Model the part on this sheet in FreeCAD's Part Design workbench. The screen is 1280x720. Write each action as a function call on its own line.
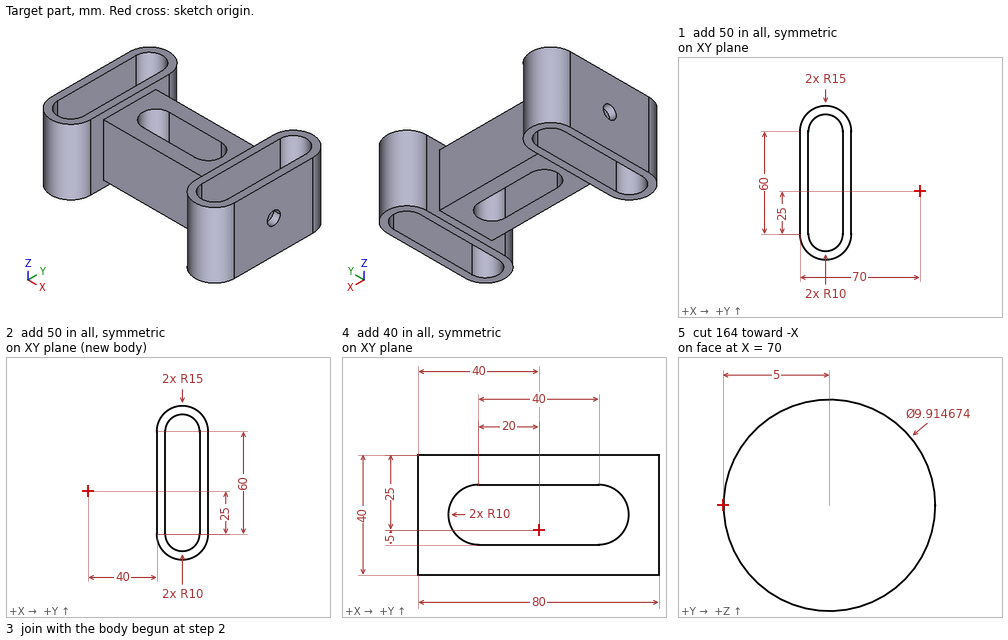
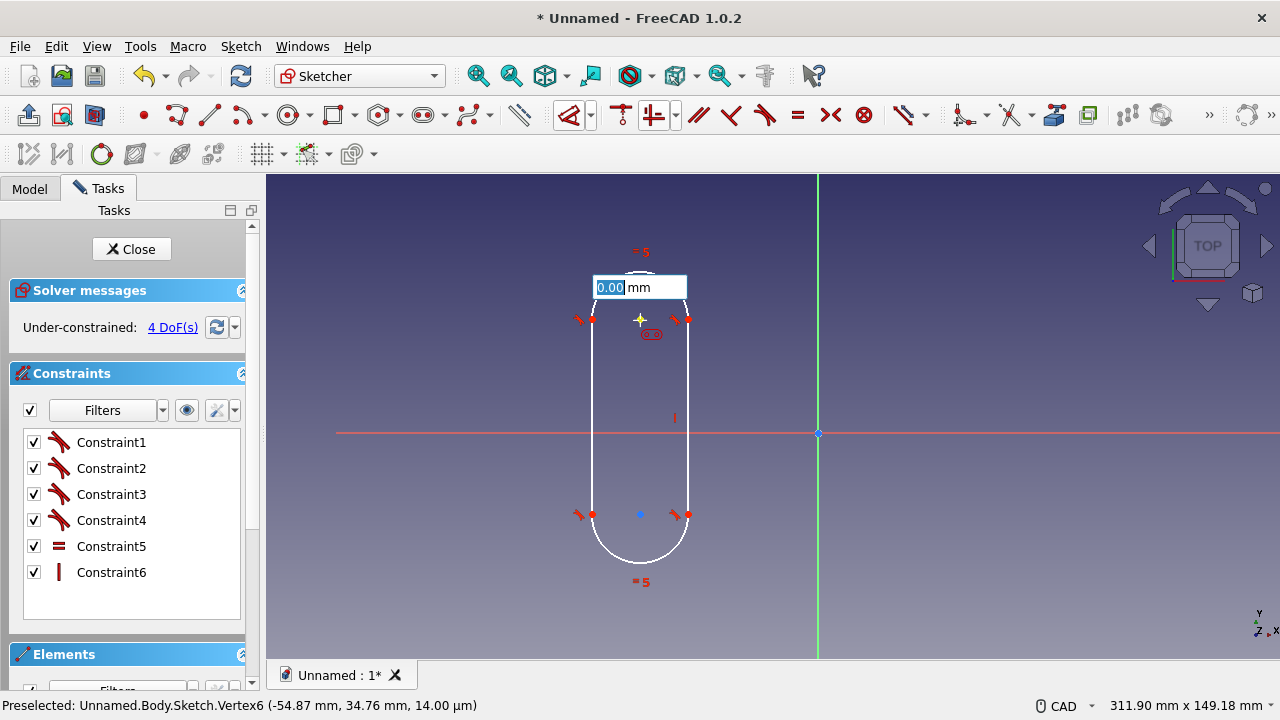
click(672, 417)
key(Escape)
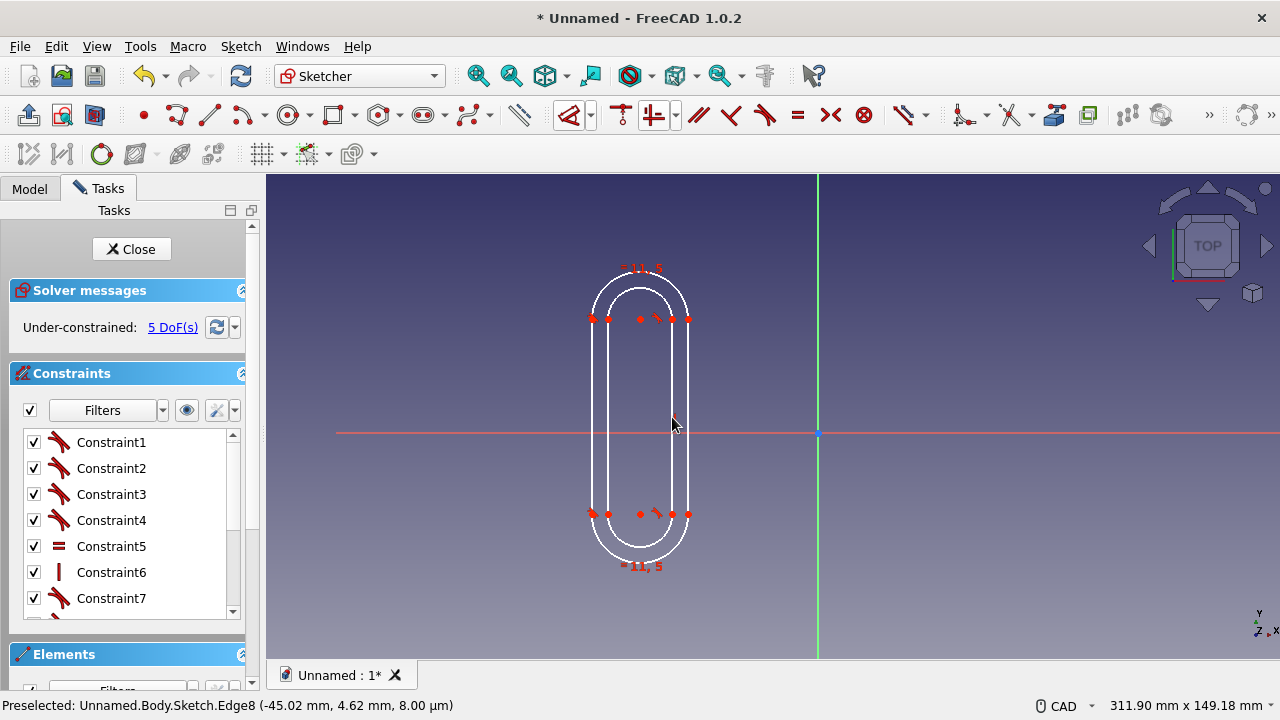
click(612, 554)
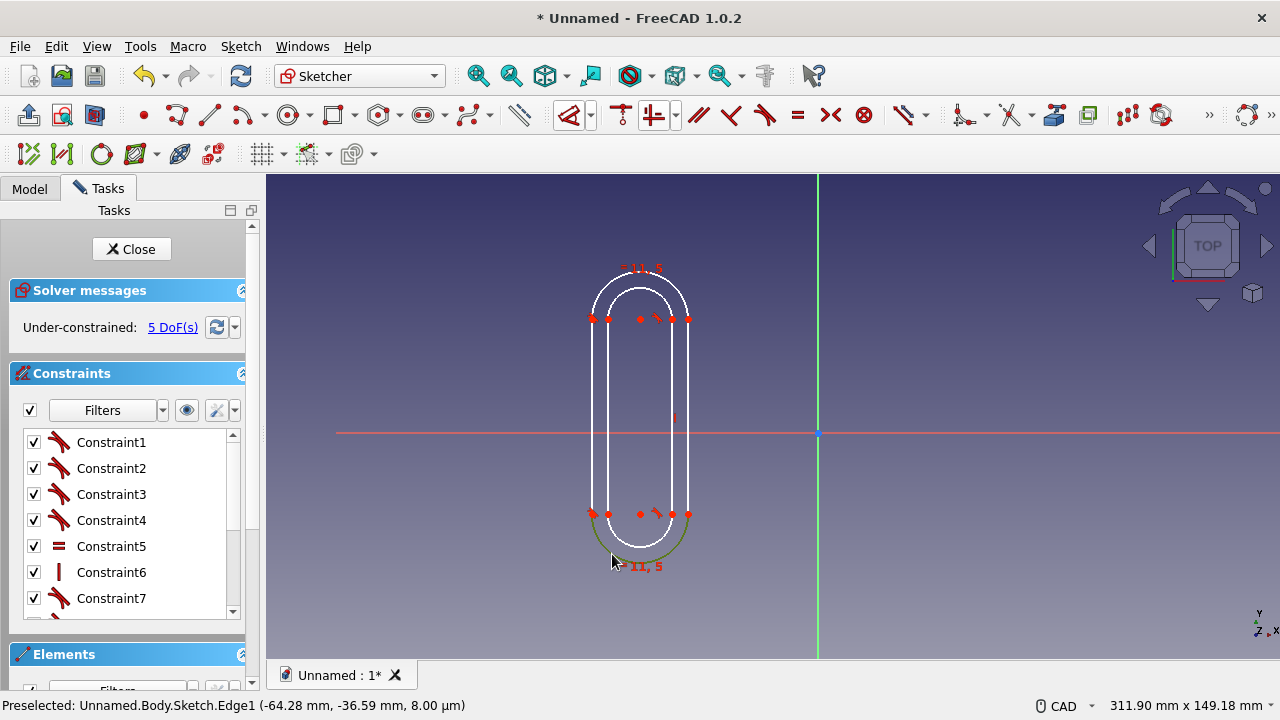
key(k)
key(r)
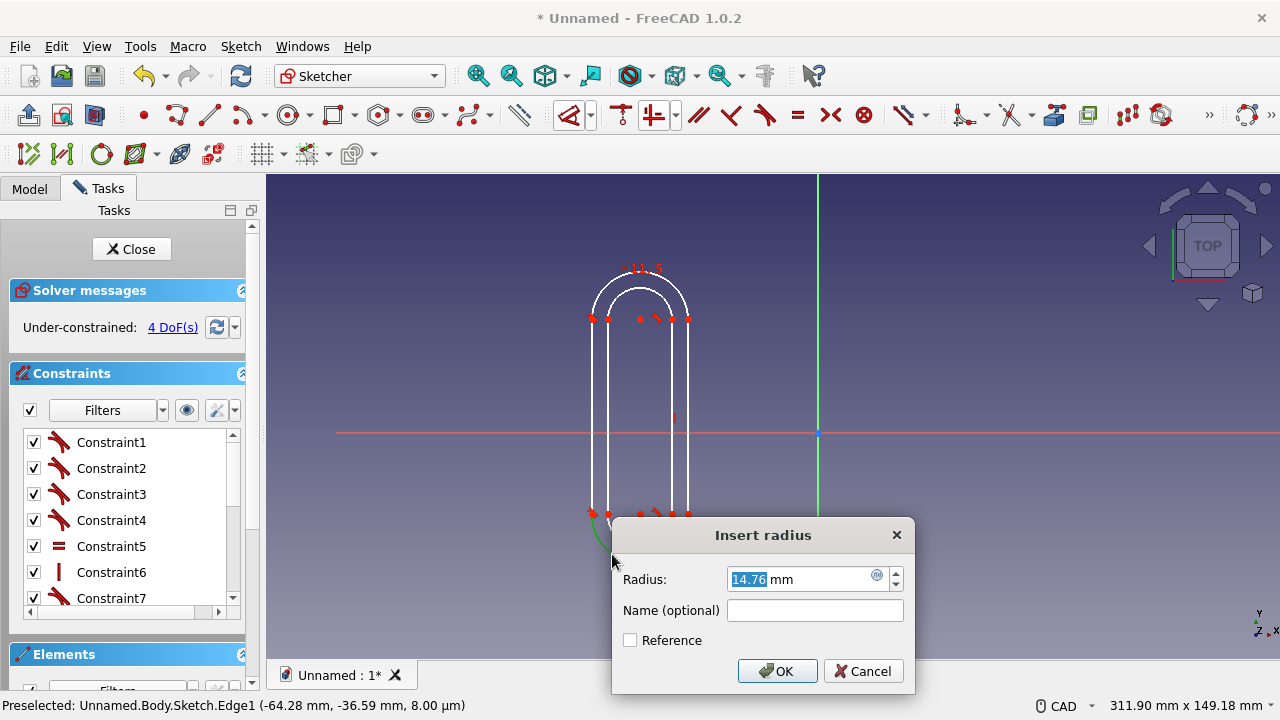
text(15)
key(Return)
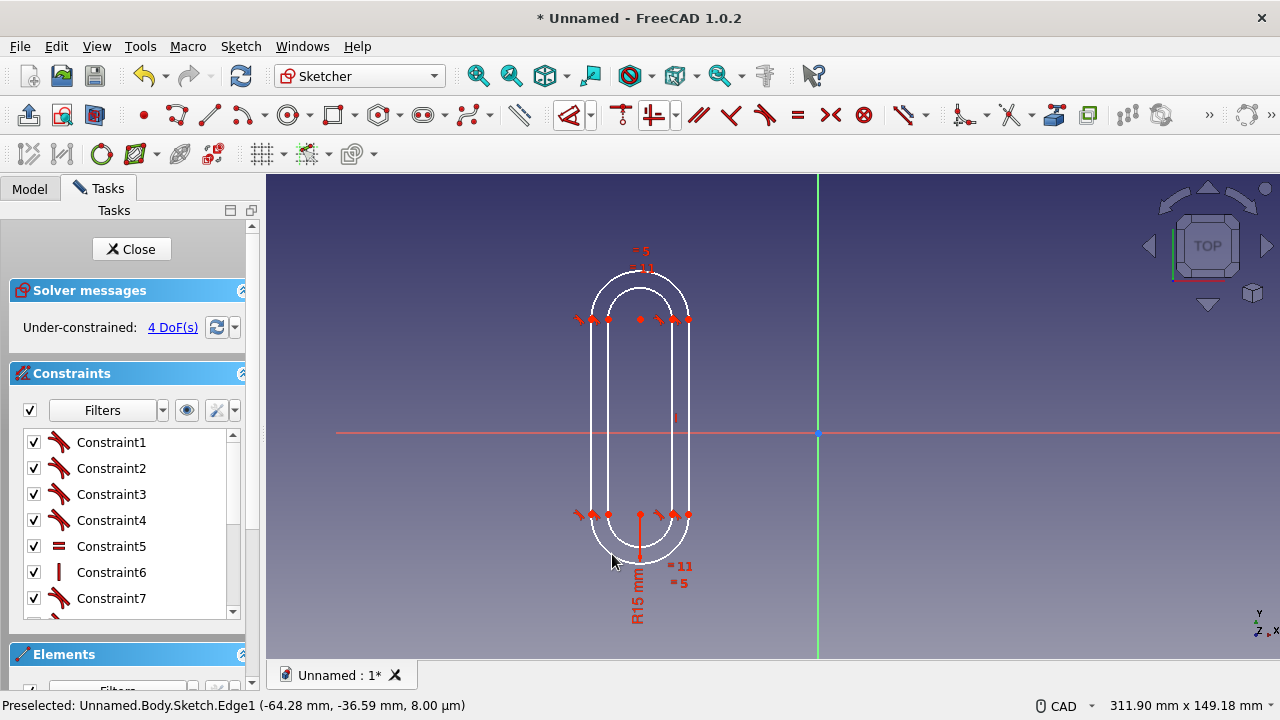
click(621, 541)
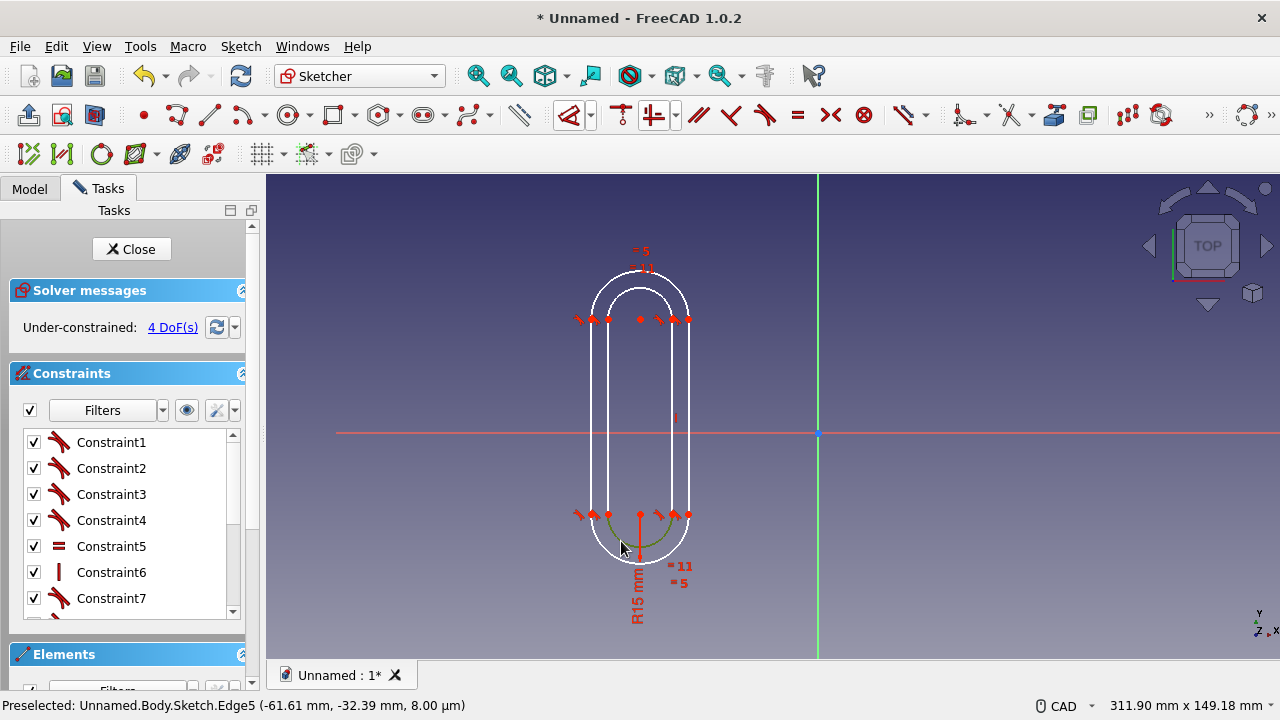
click(590, 116)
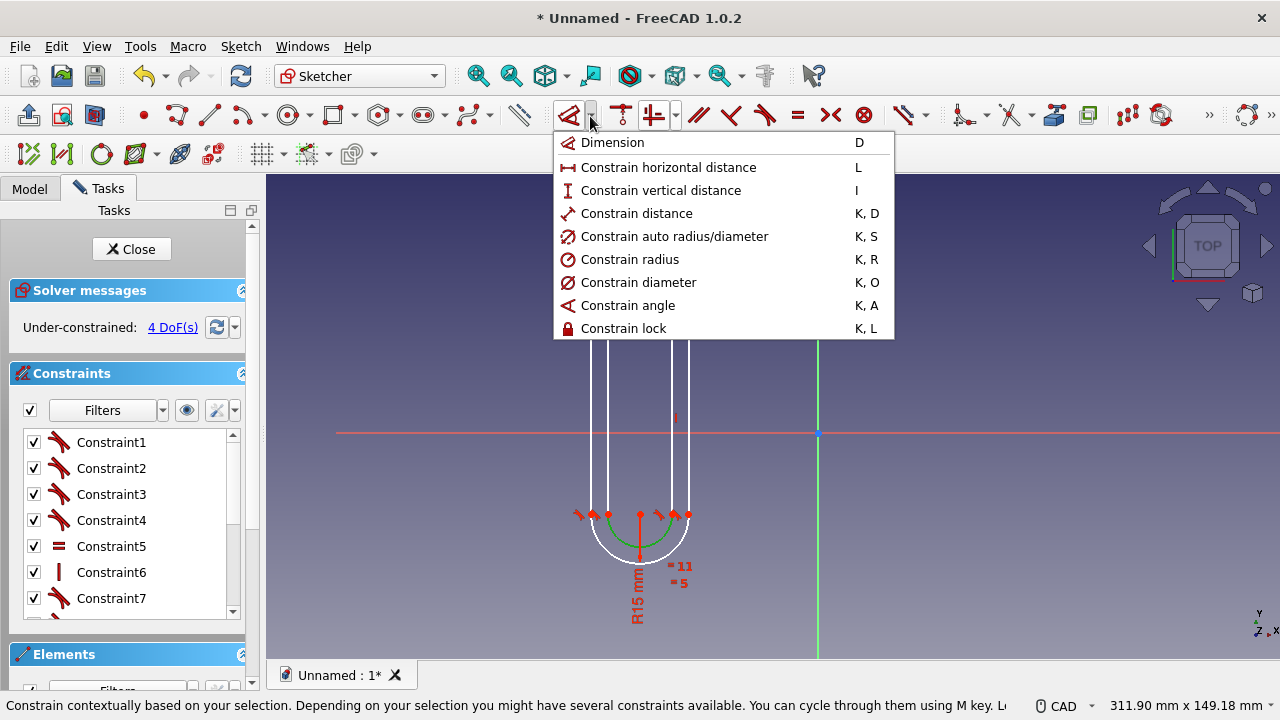
click(724, 260)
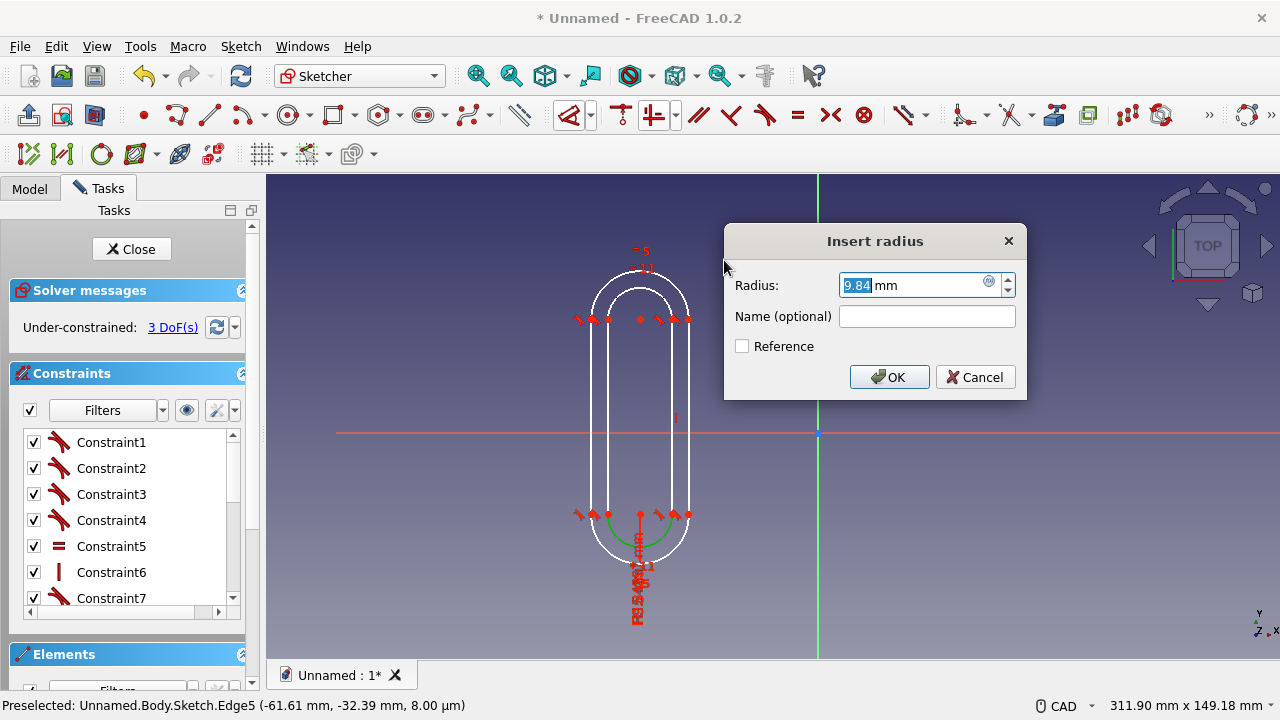
text(10)
key(Return)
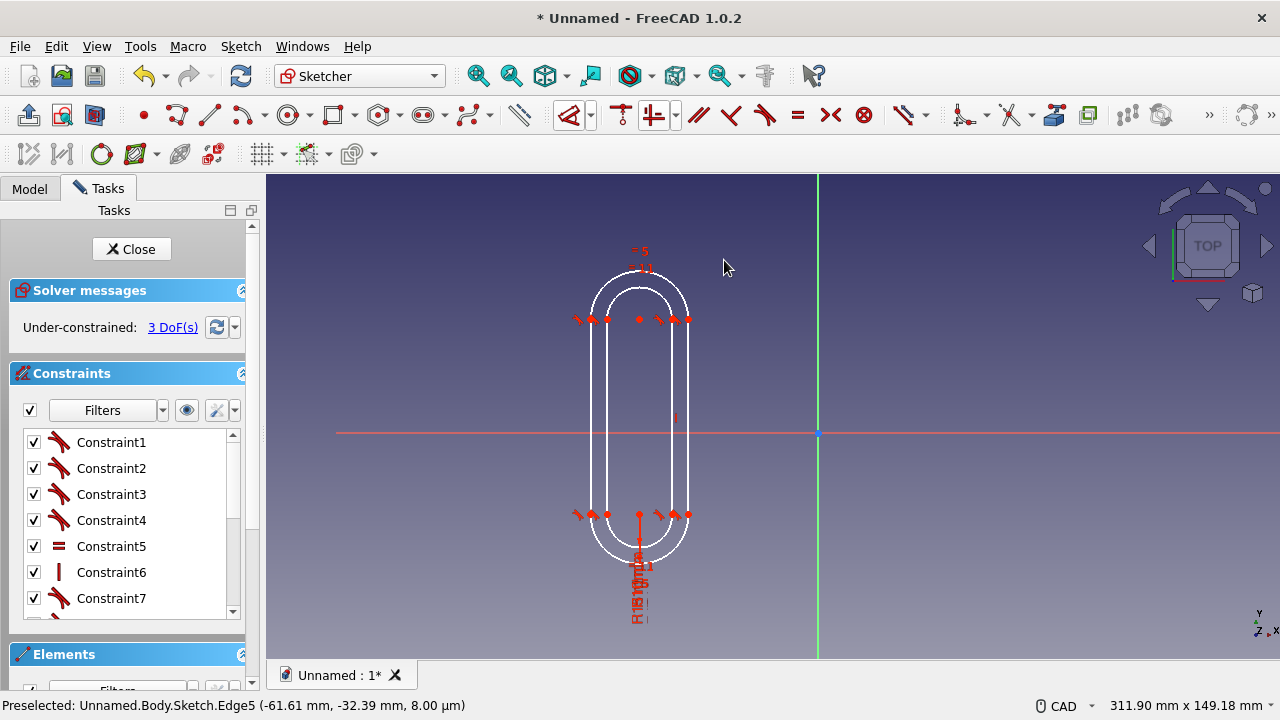
click(591, 457)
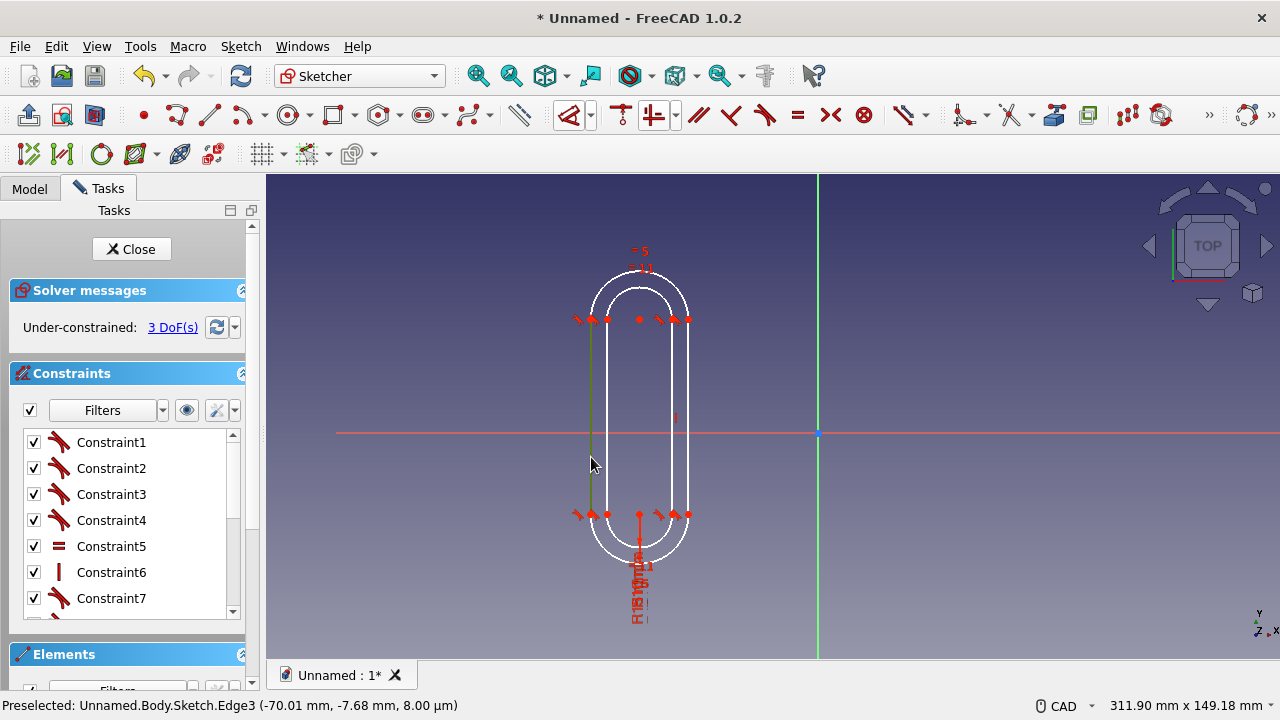
click(590, 116)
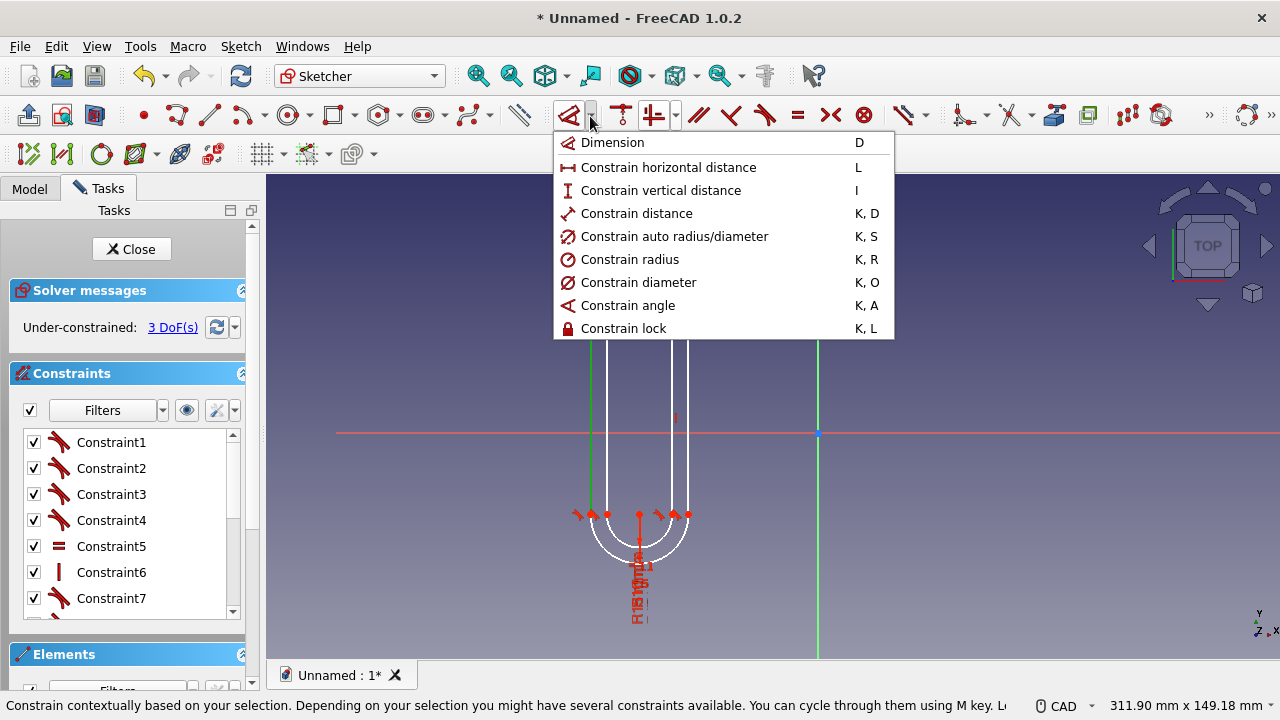
click(724, 190)